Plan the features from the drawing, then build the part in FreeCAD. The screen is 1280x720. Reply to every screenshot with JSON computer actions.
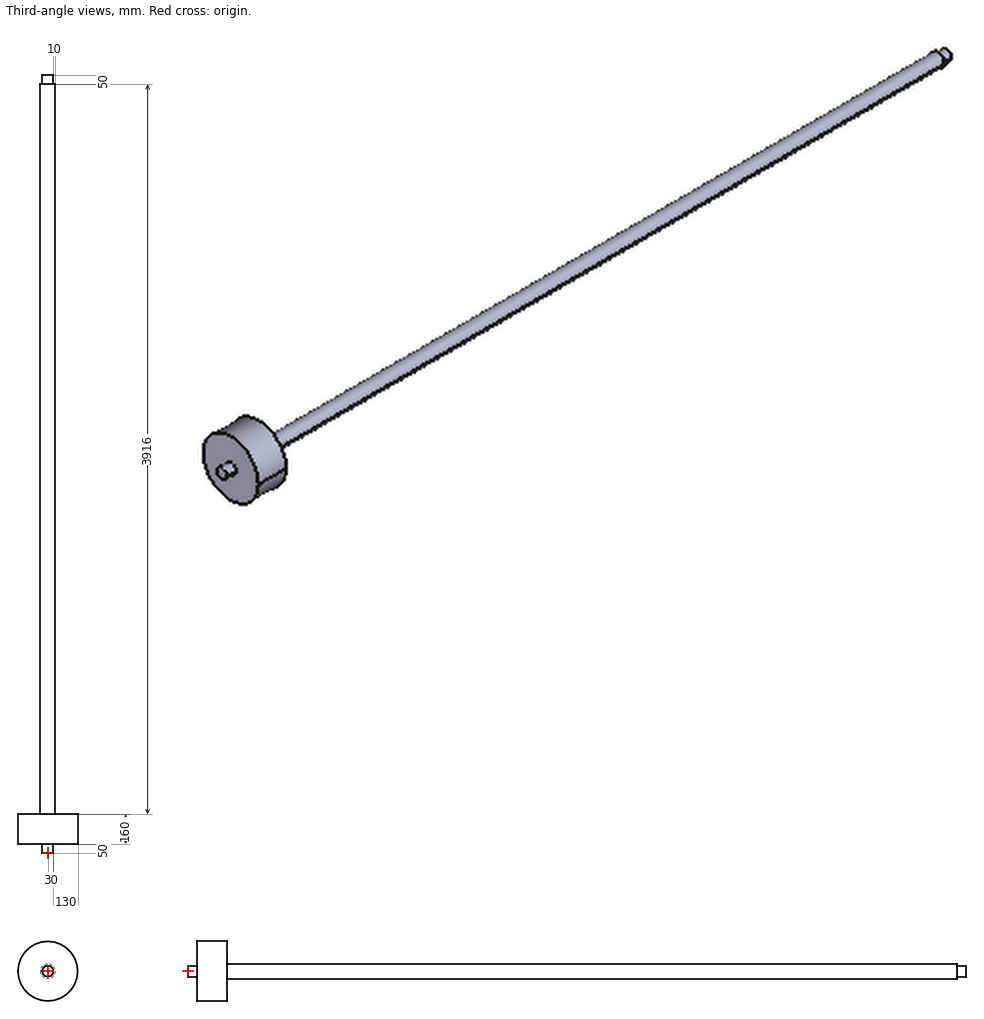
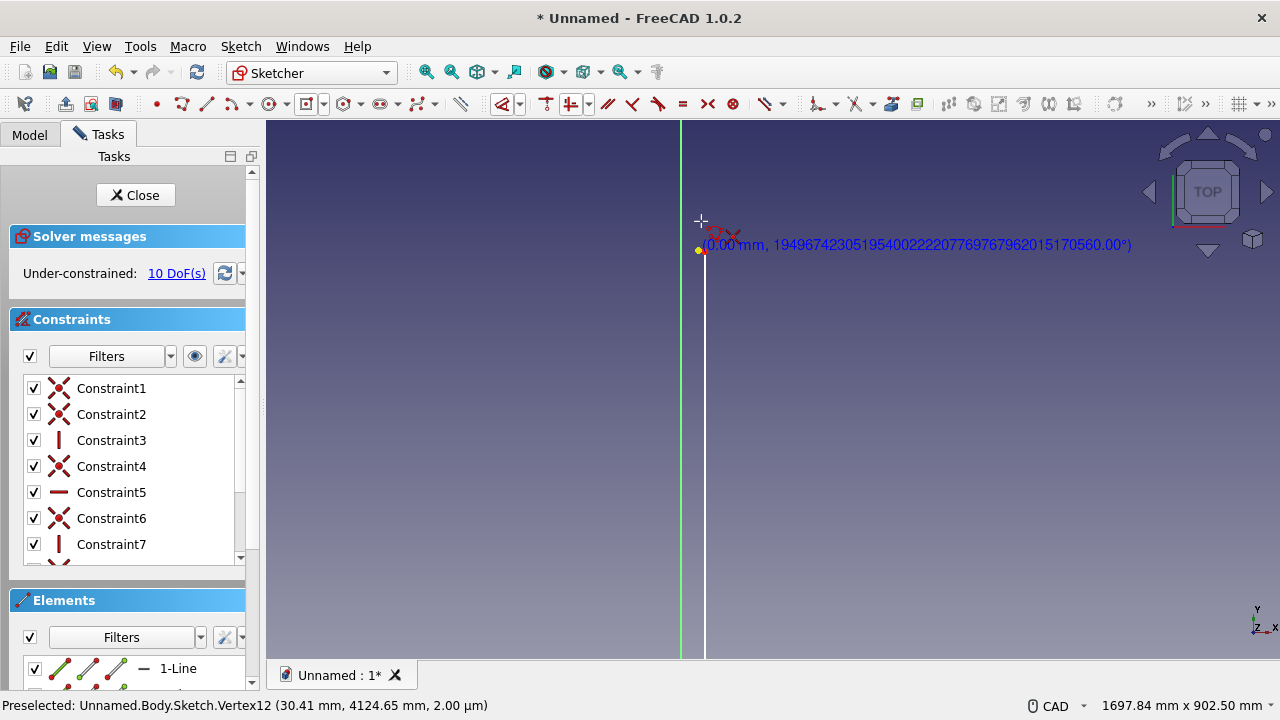
{"action": "left_click", "coordinate": [698, 220]}
{"action": "left_click", "coordinate": [690, 220]}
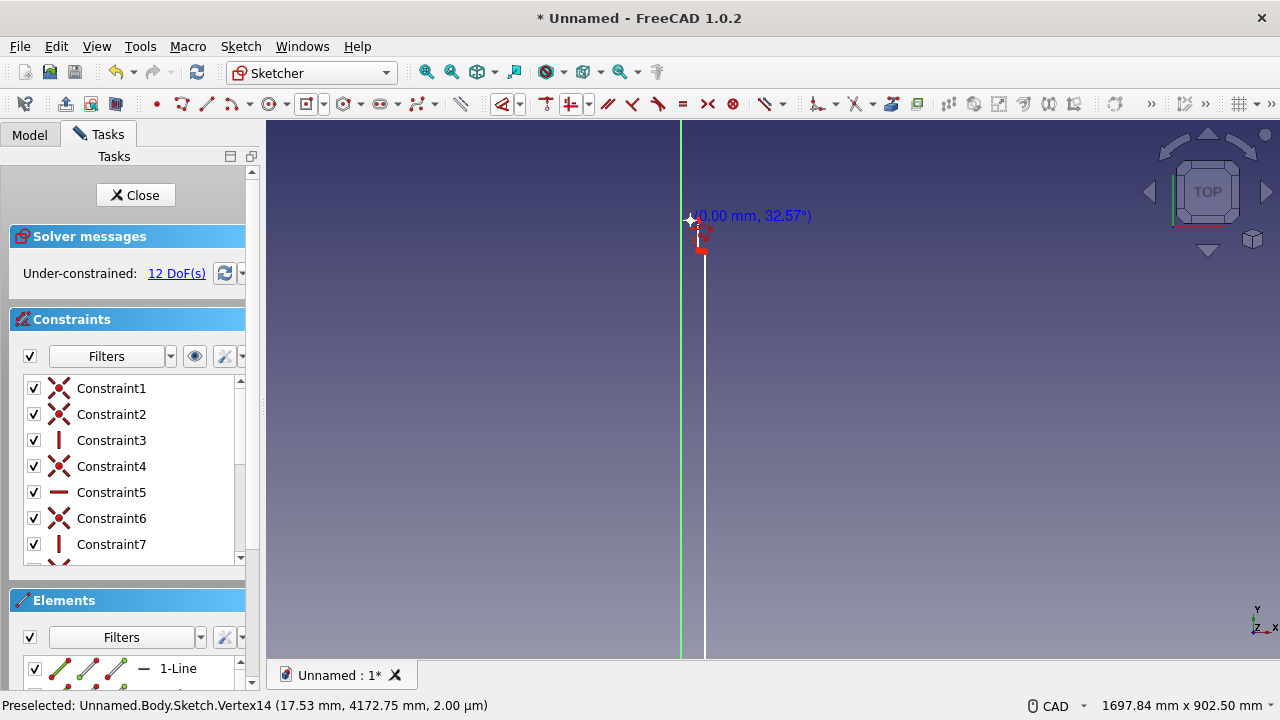
{"action": "scroll", "coordinate": [701, 221], "scroll_direction": "down", "scroll_amount": 10}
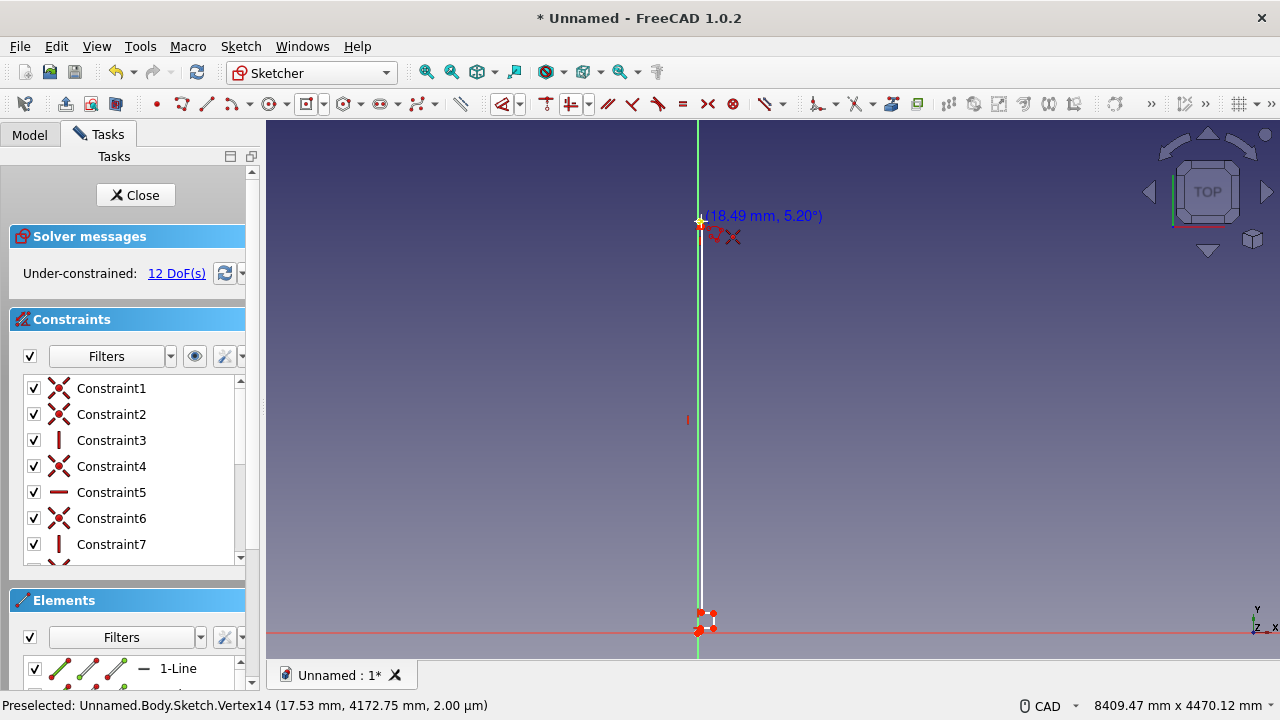
{"action": "scroll", "coordinate": [699, 559], "scroll_direction": "up", "scroll_amount": 13}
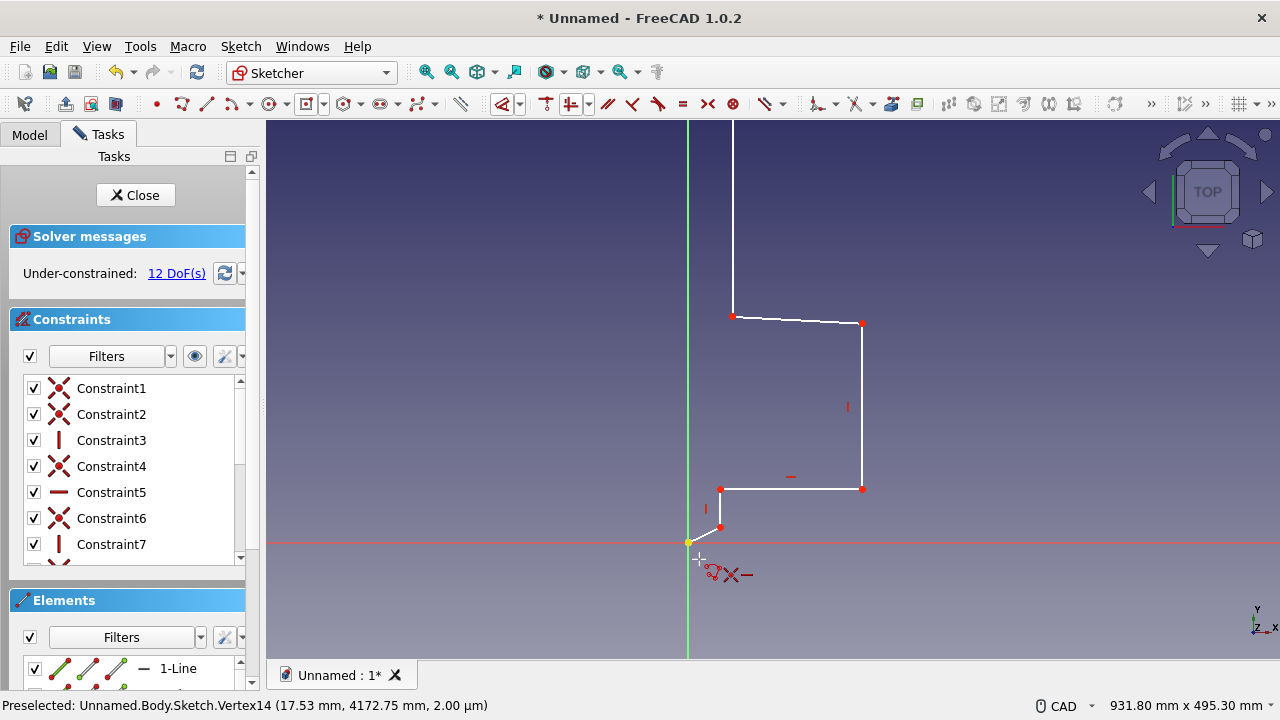
{"action": "left_click", "coordinate": [688, 543]}
{"action": "key", "text": "Escape"}
{"action": "key", "text": "Escape"}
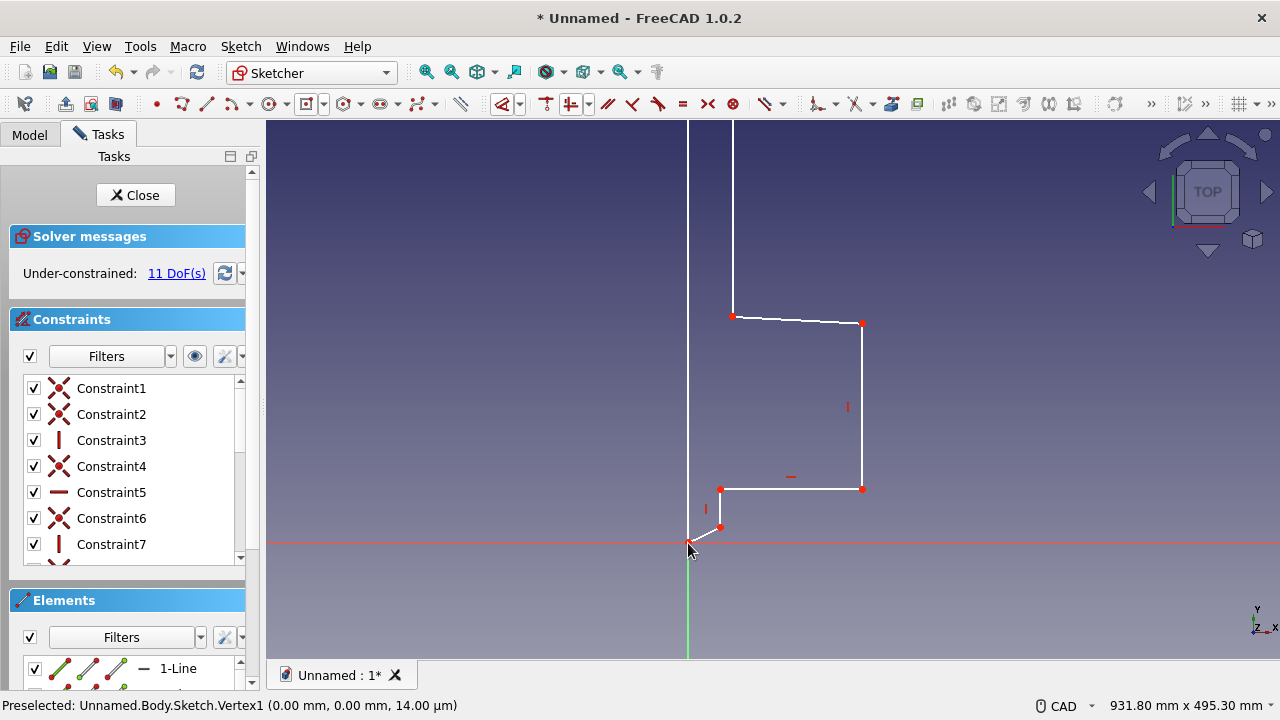
{"action": "left_click", "coordinate": [711, 532]}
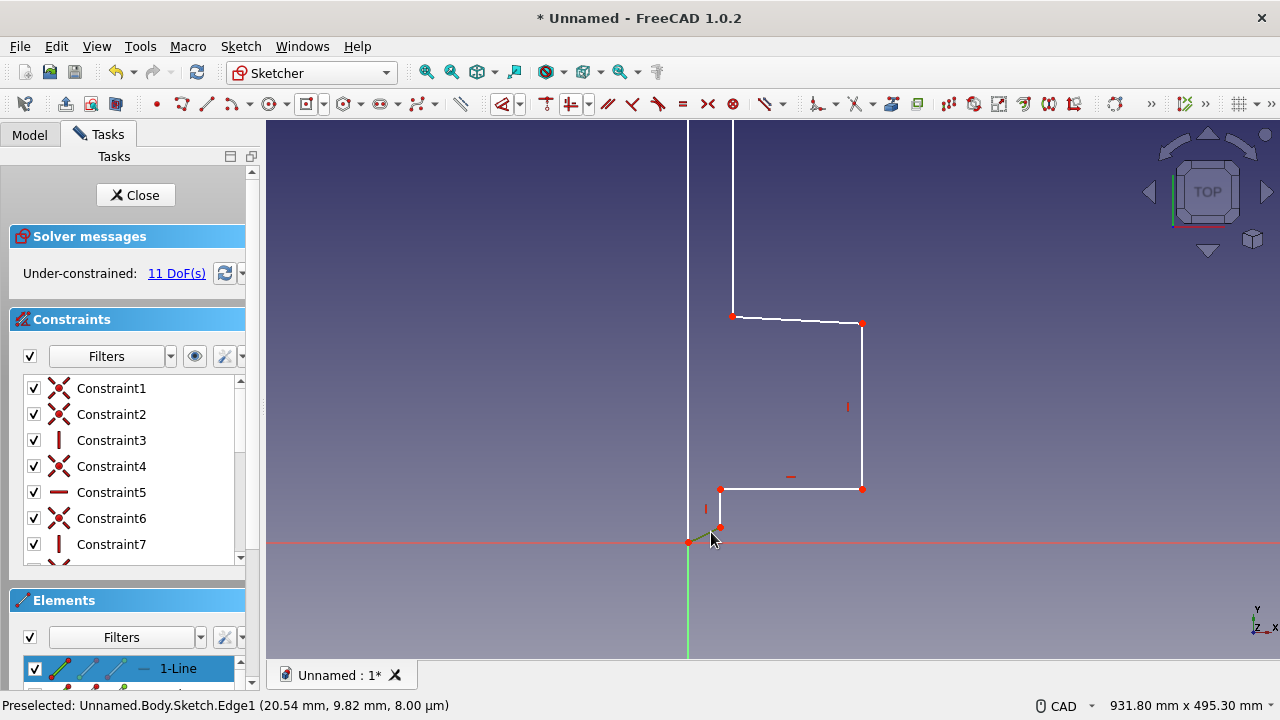
{"action": "left_click", "coordinate": [588, 104]}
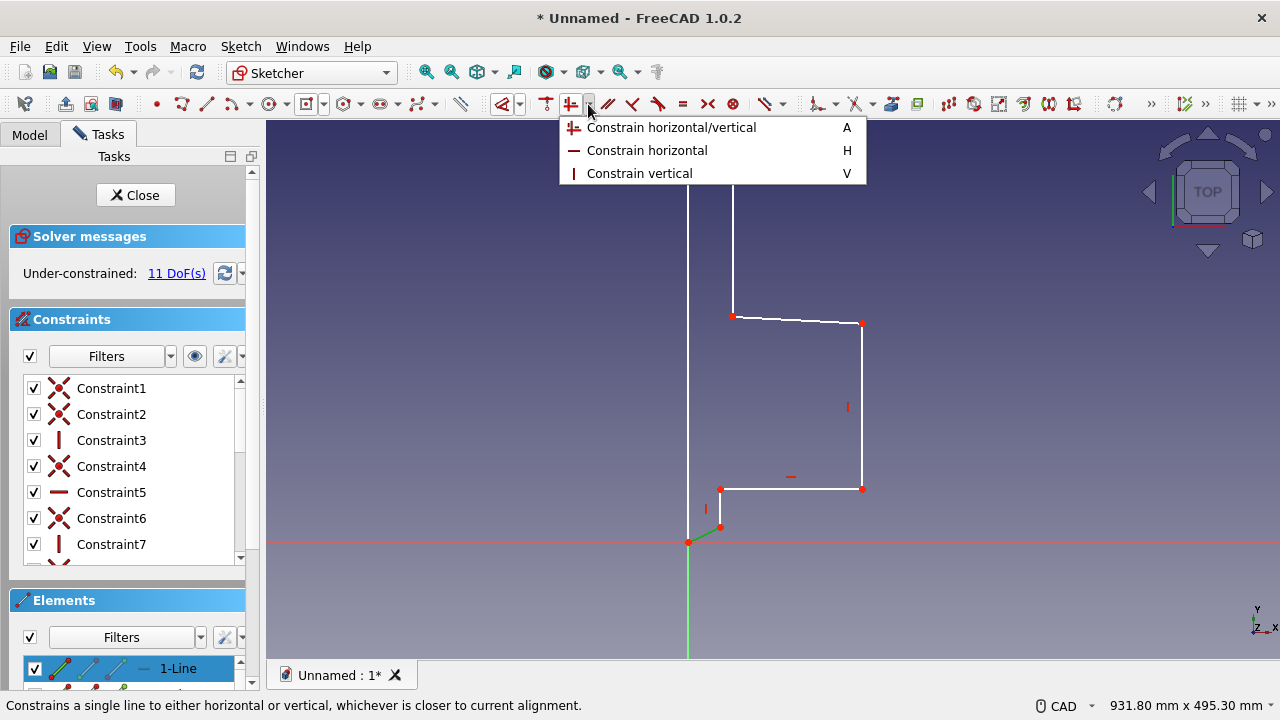
{"action": "left_click", "coordinate": [713, 150]}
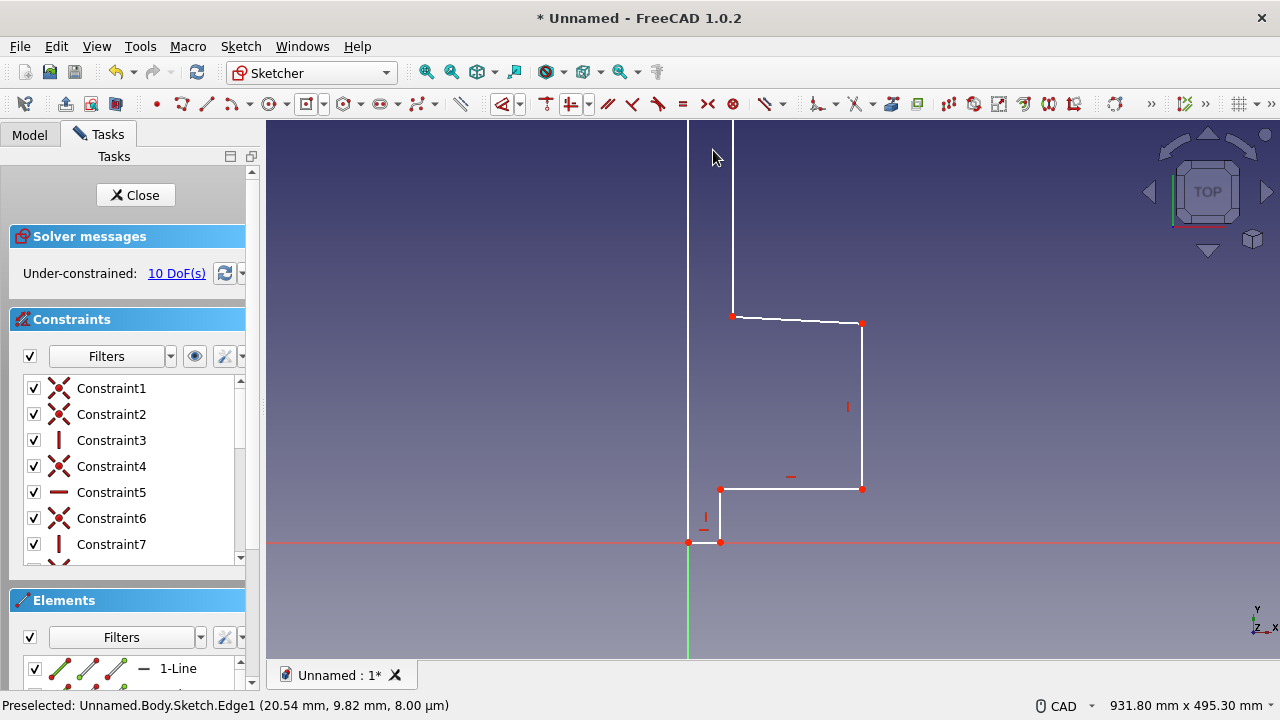
{"action": "left_click", "coordinate": [823, 322]}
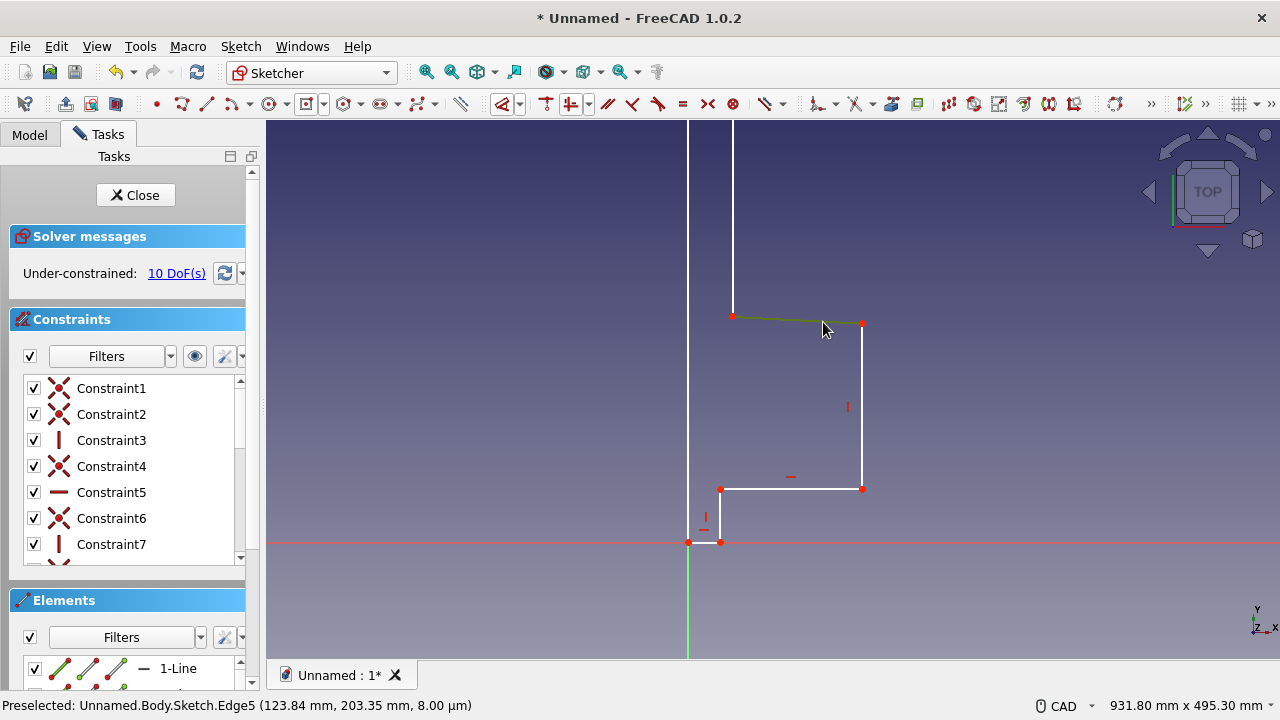
{"action": "key", "text": "h"}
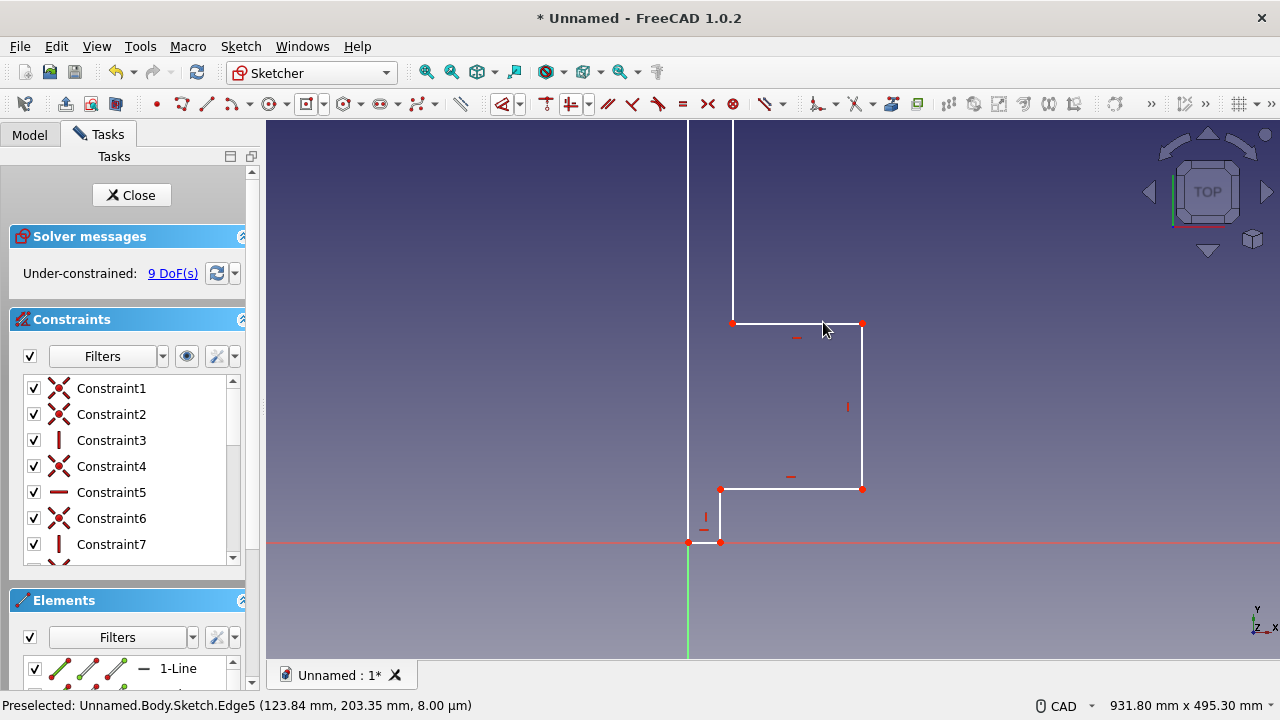
{"action": "scroll", "coordinate": [699, 559], "scroll_direction": "down", "scroll_amount": 13}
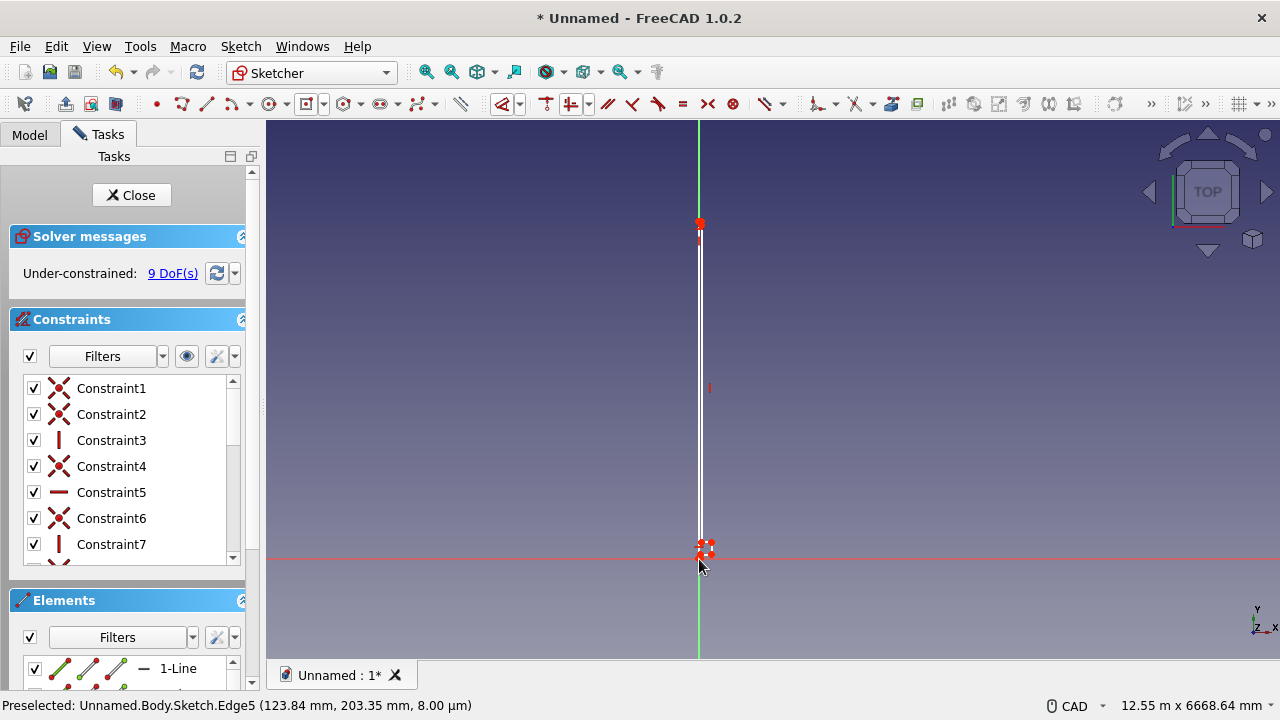
{"action": "scroll", "coordinate": [701, 225], "scroll_direction": "up", "scroll_amount": 14}